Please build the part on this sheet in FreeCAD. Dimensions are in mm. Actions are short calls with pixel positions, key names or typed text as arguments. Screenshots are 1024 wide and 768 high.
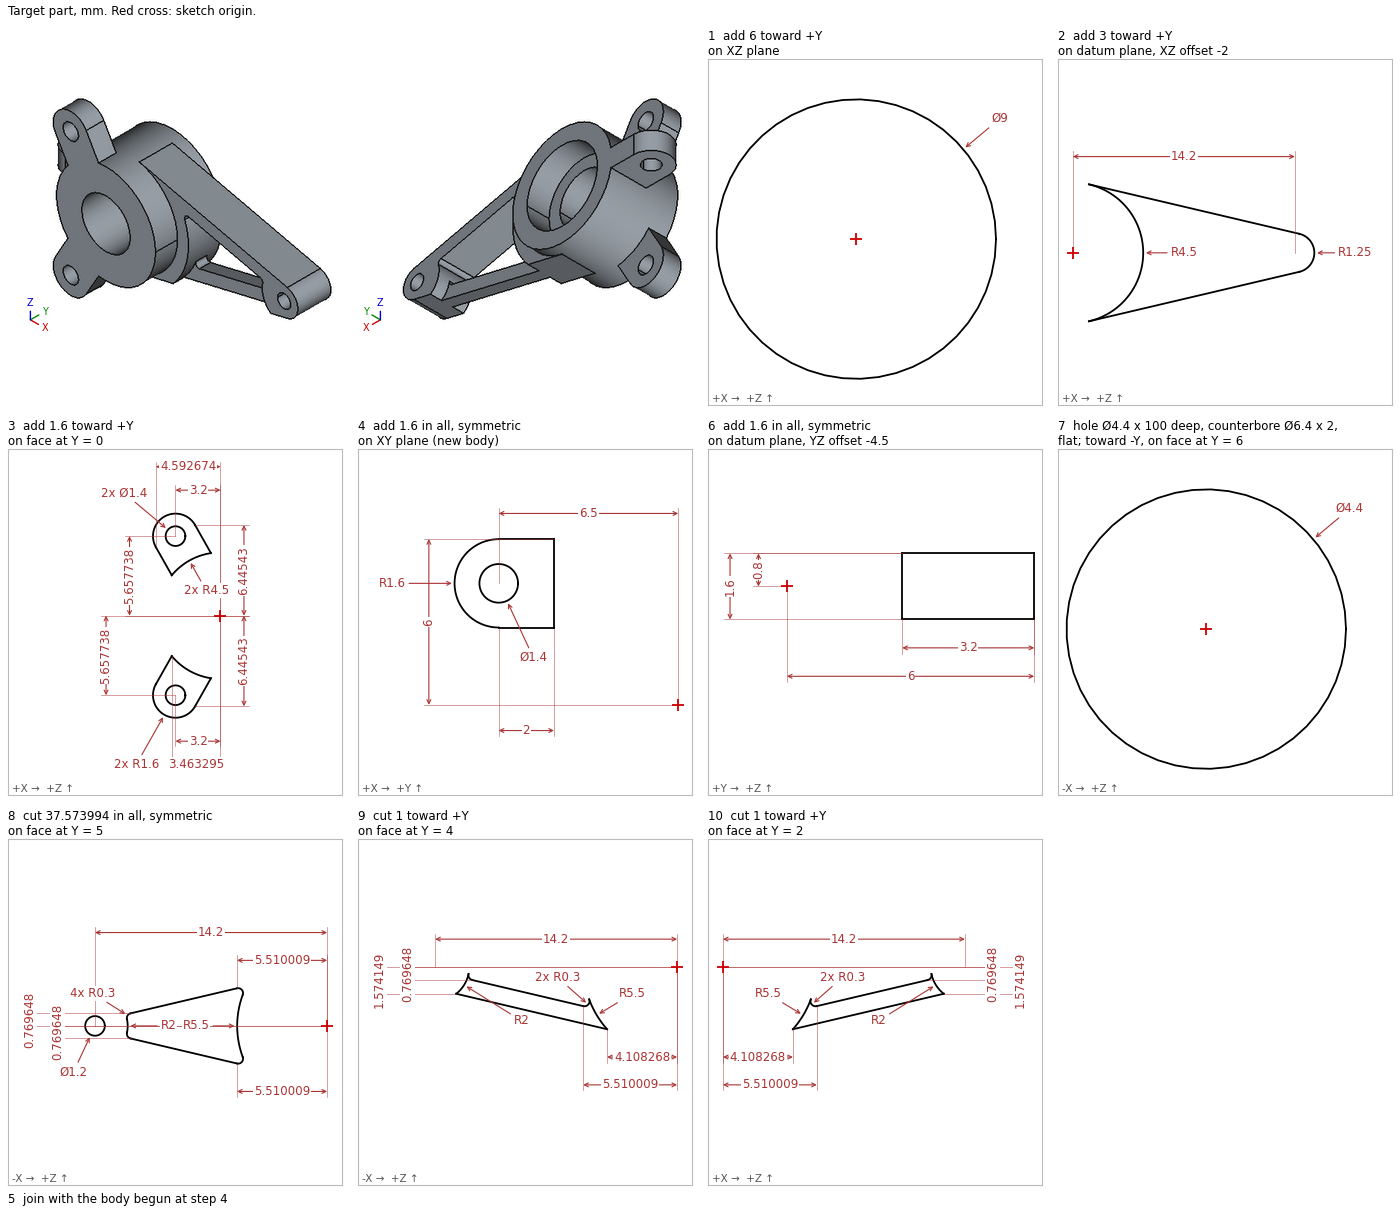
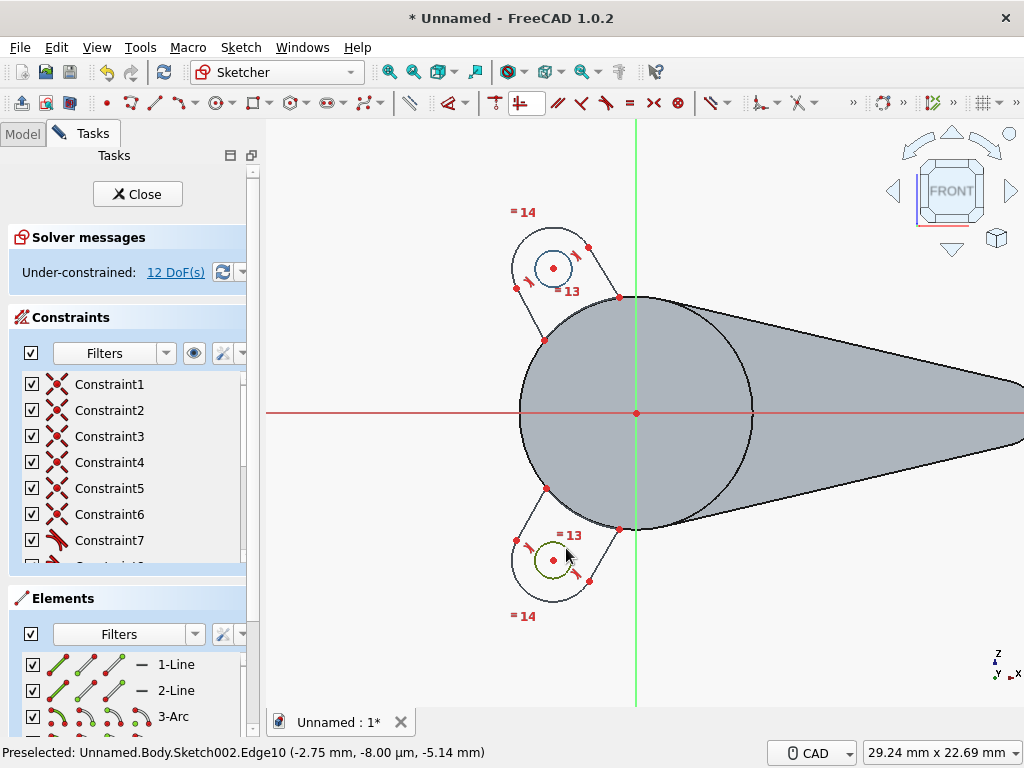
key(e)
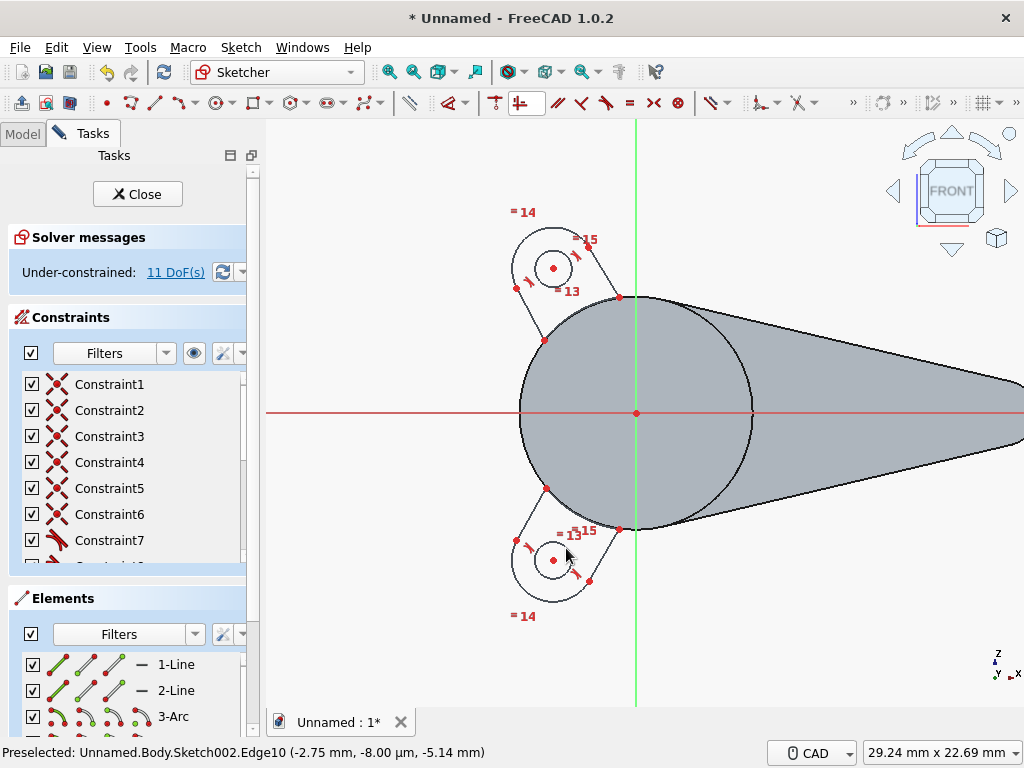
click(448, 104)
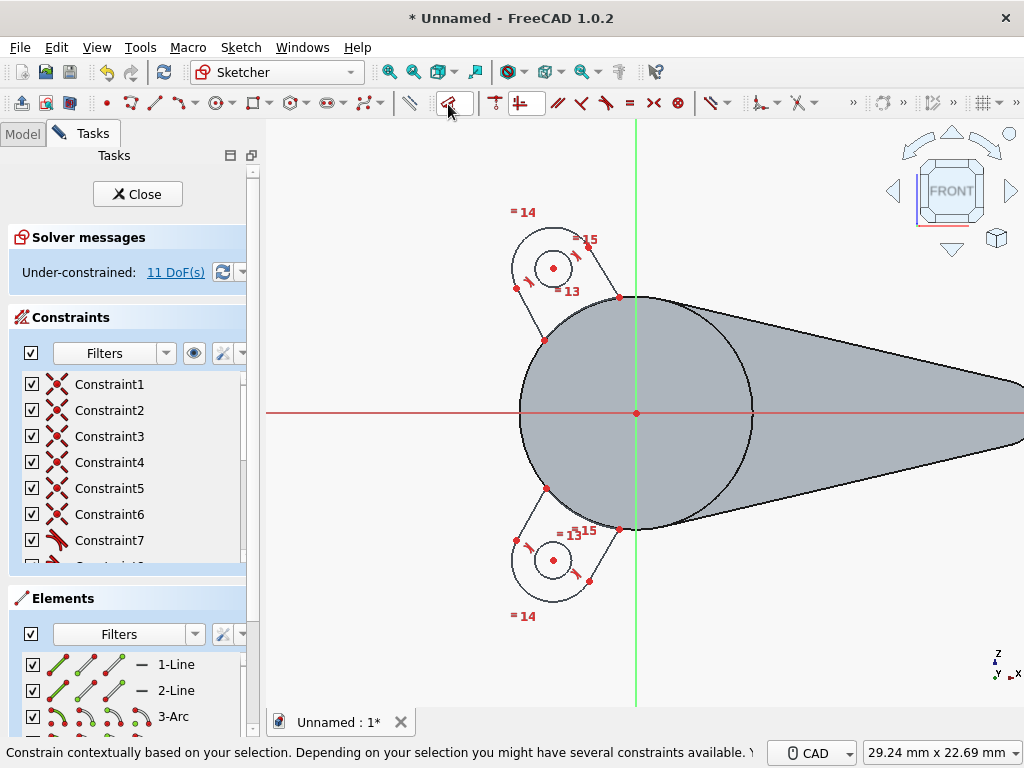
click(558, 228)
click(561, 196)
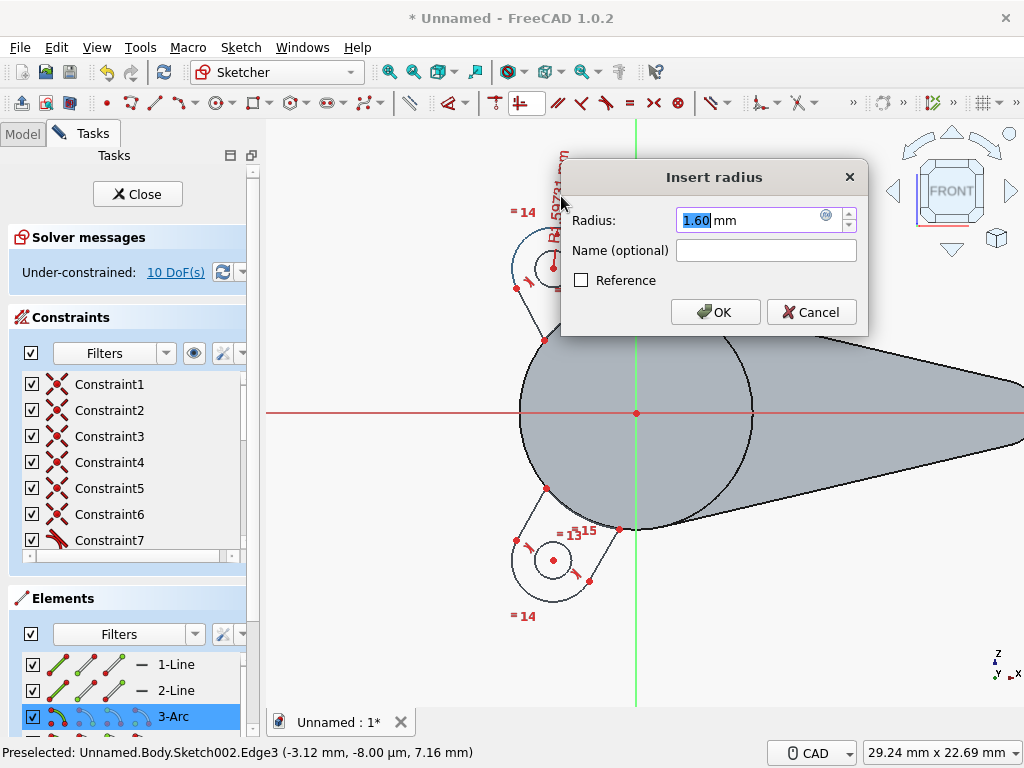
text(1.6)
key(Return)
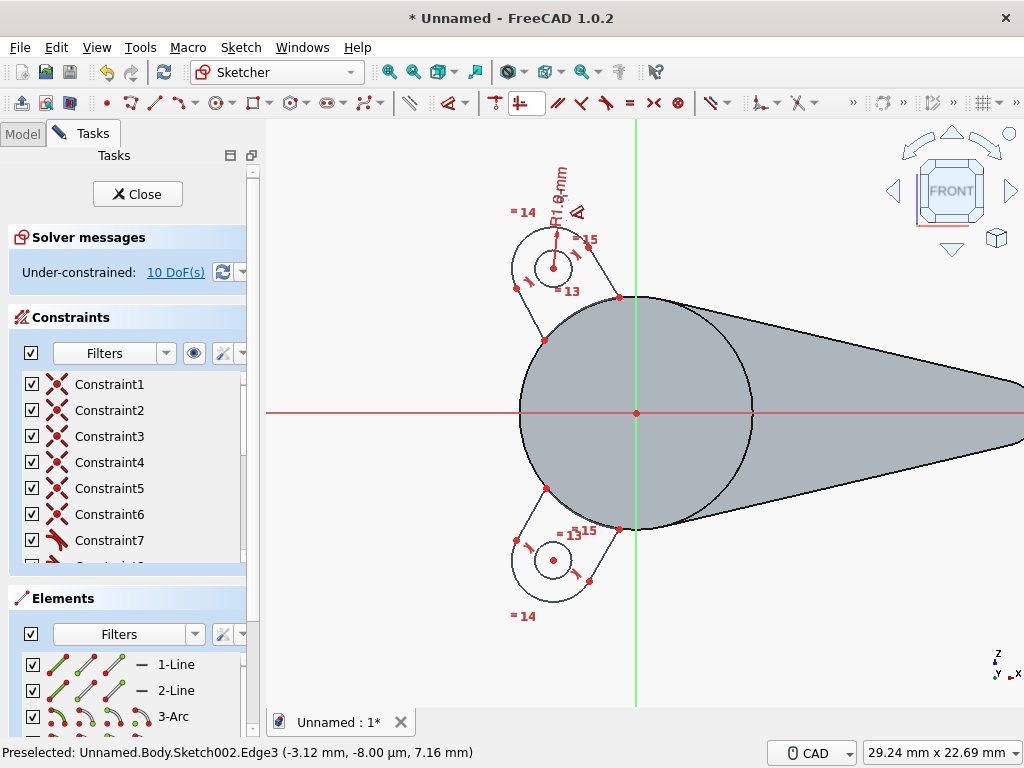
click(594, 304)
click(656, 265)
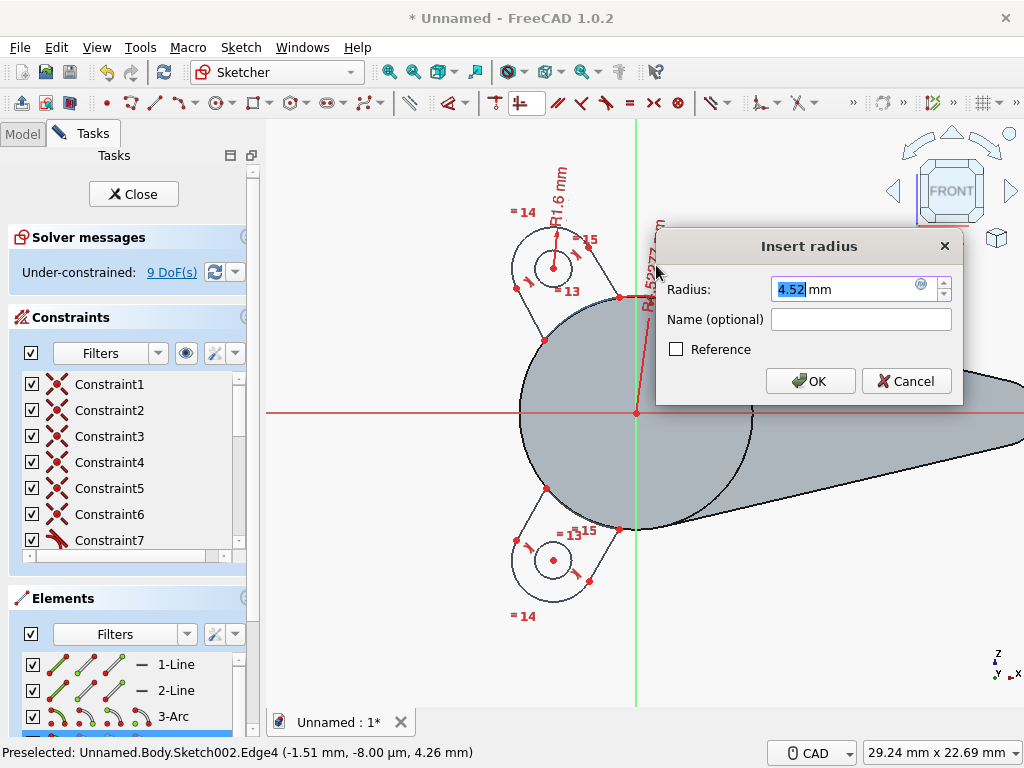
text(4.5)
key(Return)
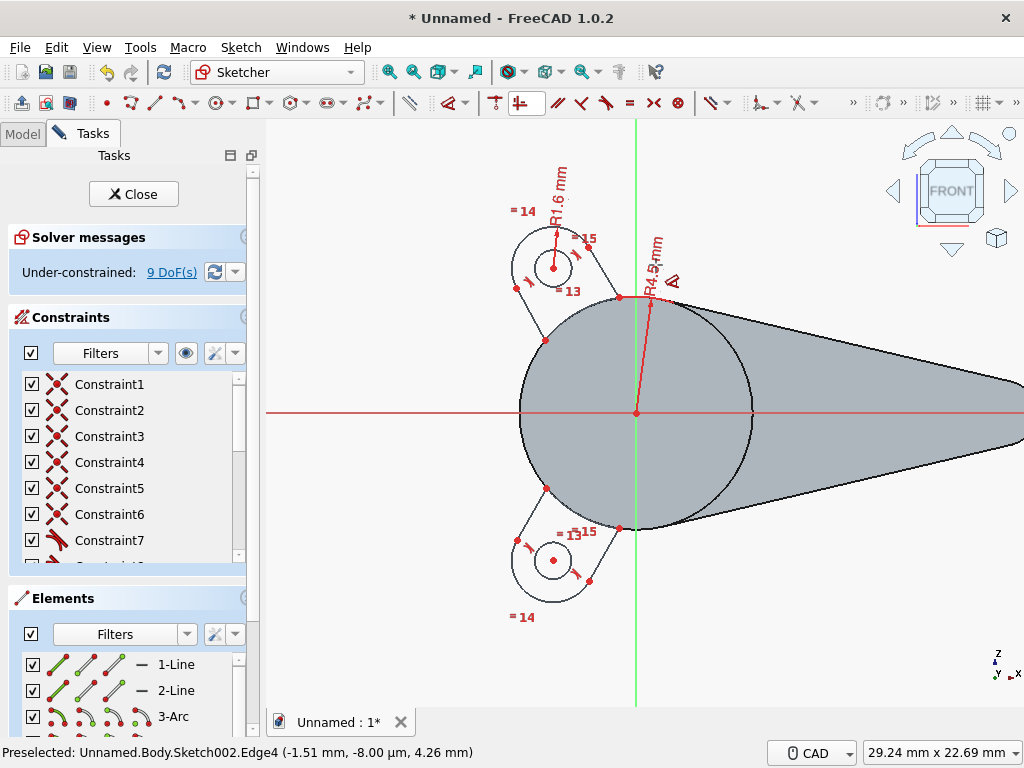
click(566, 255)
click(607, 319)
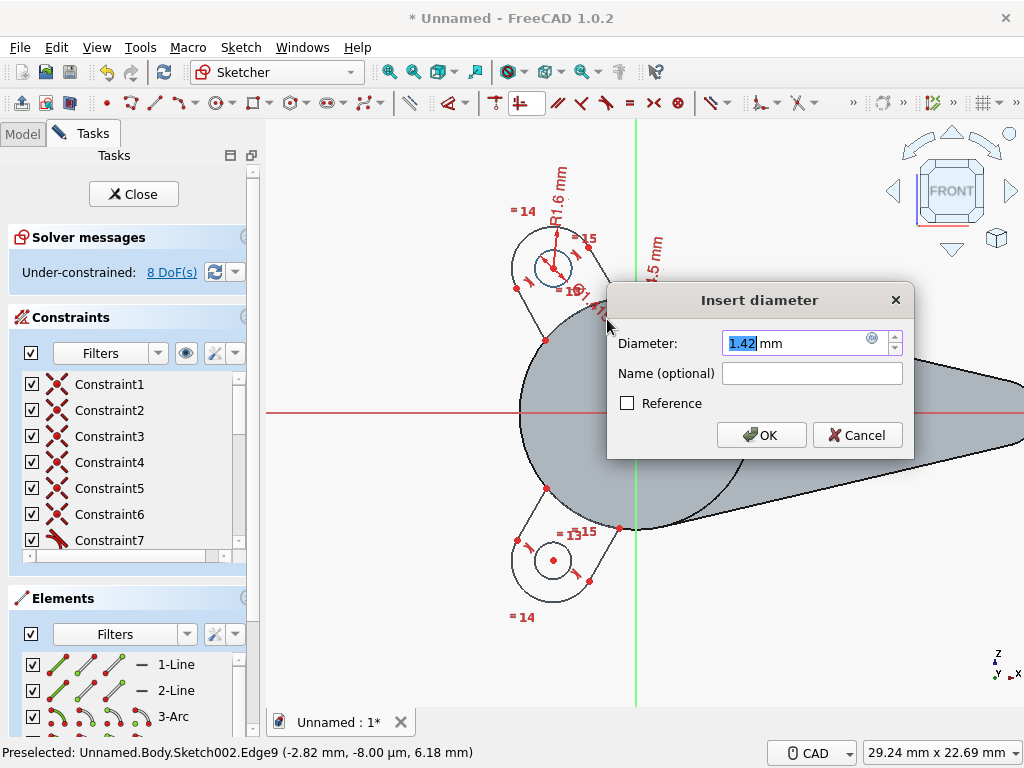
text(1.4)
key(Return)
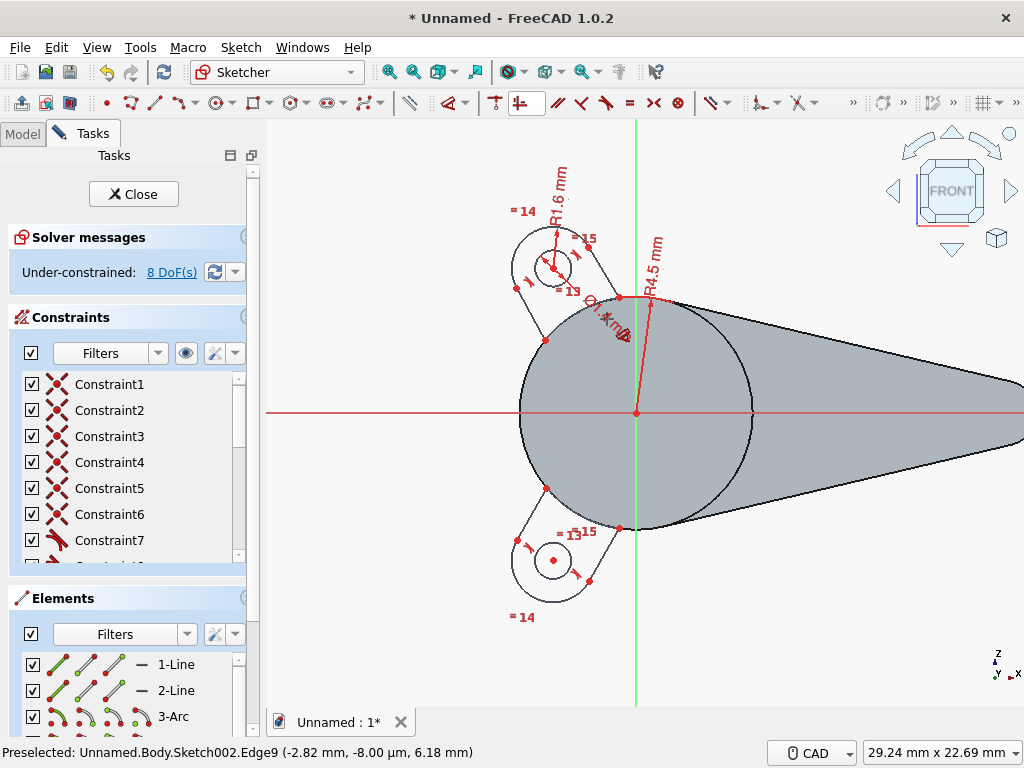
click(553, 268)
click(614, 234)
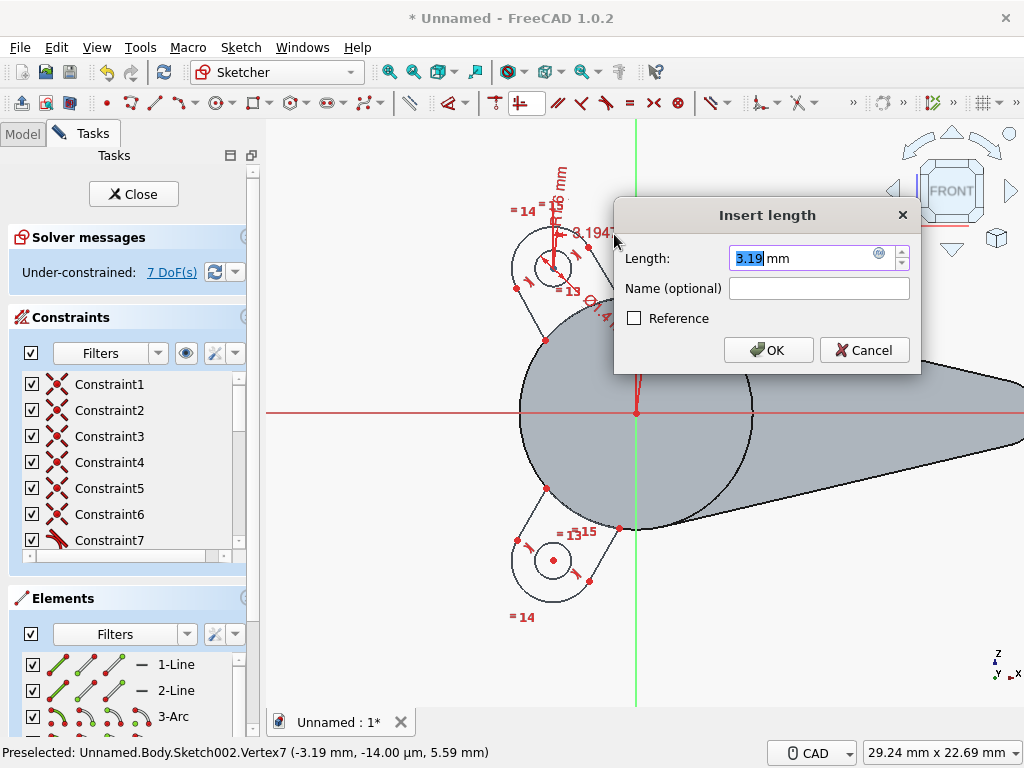
text(3.2)
key(Return)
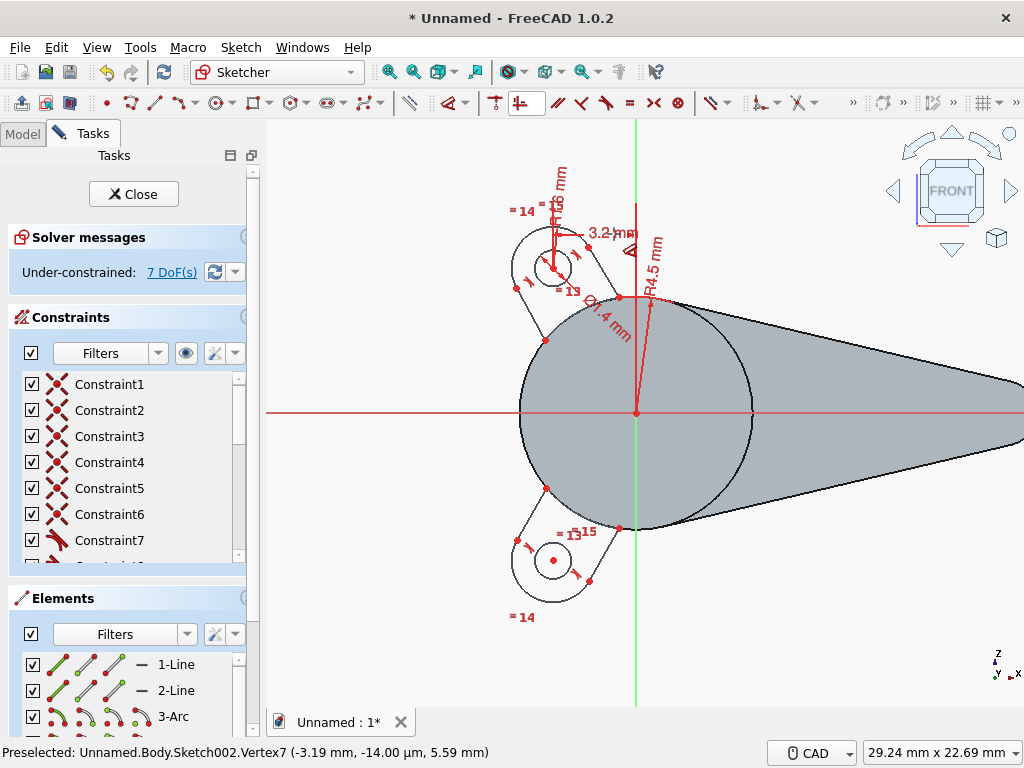
click(553, 561)
click(614, 595)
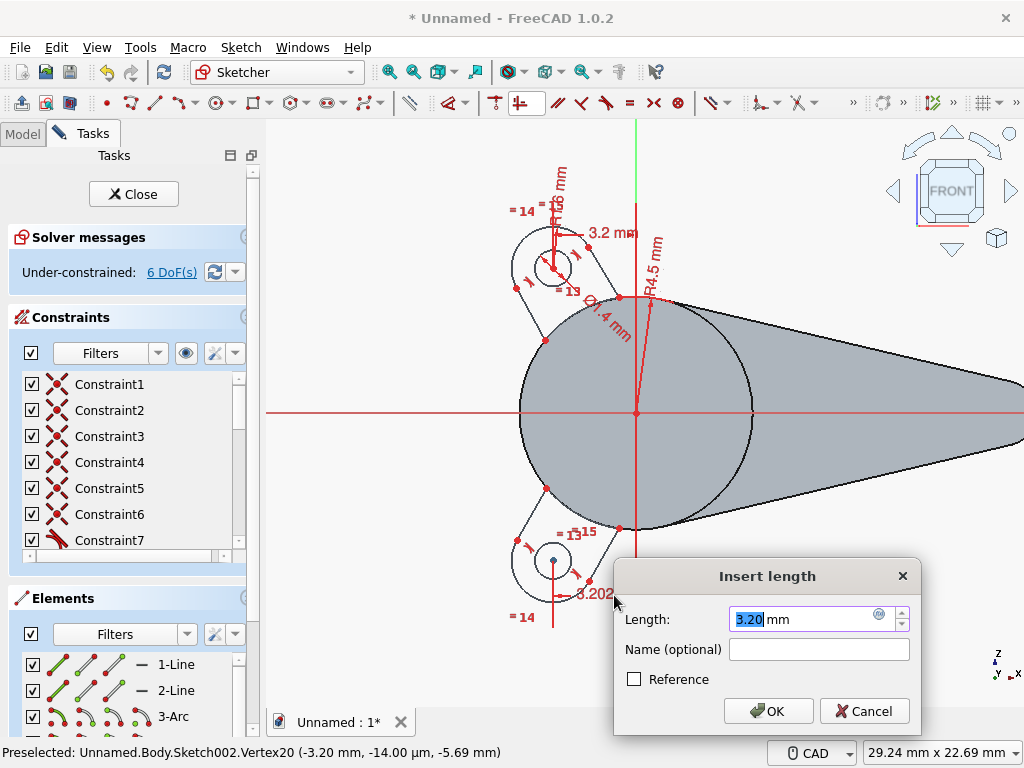
text(3.2)
key(Return)